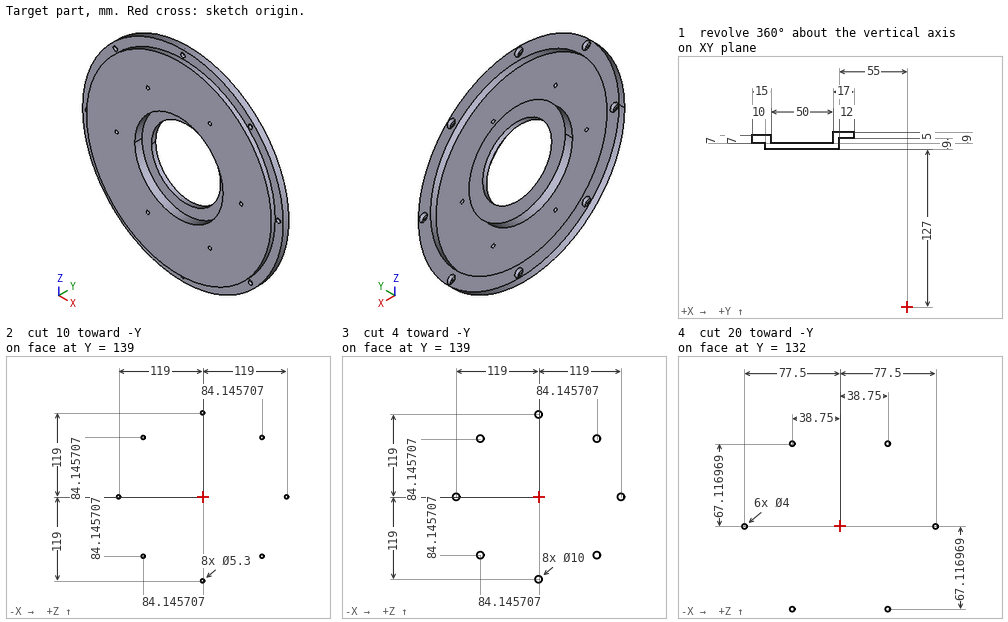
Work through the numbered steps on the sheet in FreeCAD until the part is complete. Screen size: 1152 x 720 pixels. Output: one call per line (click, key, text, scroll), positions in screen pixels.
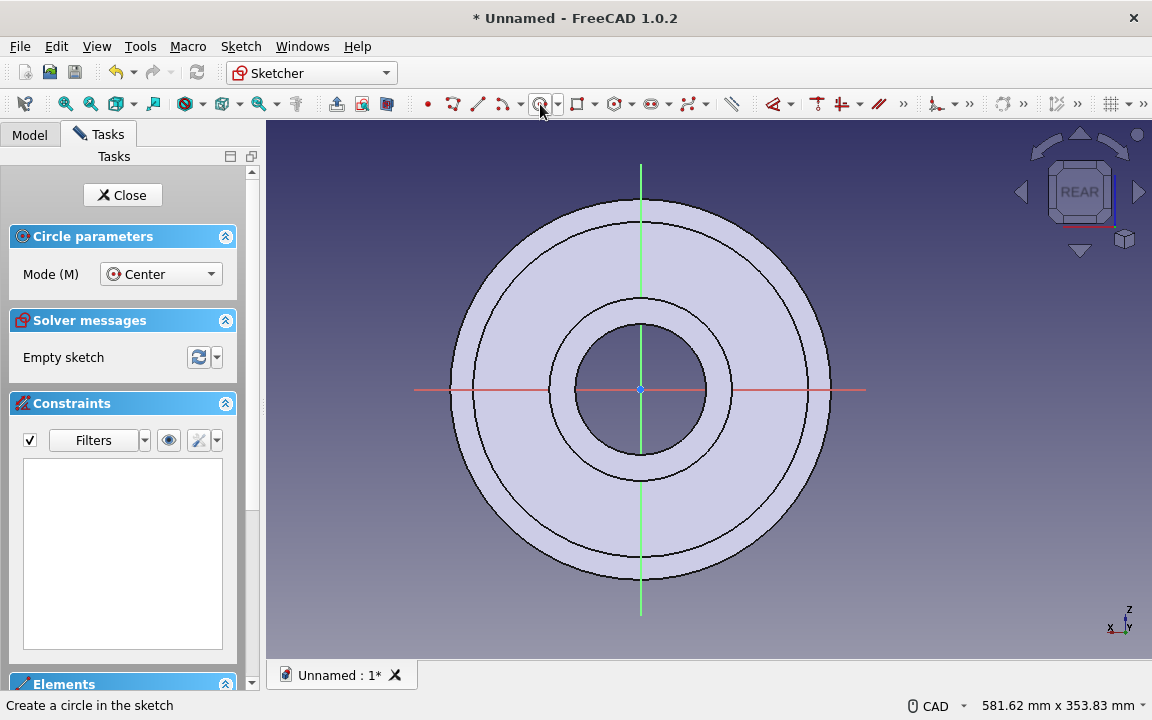
scroll(641, 571, up, 9)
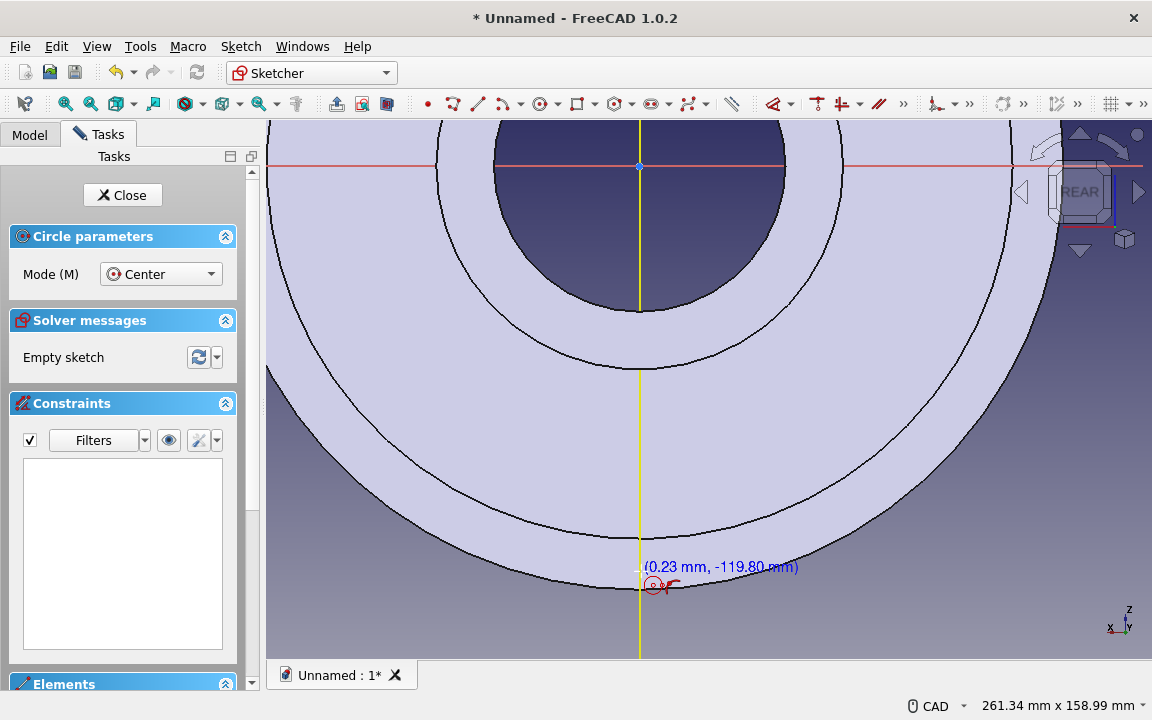
scroll(641, 572, down, 9)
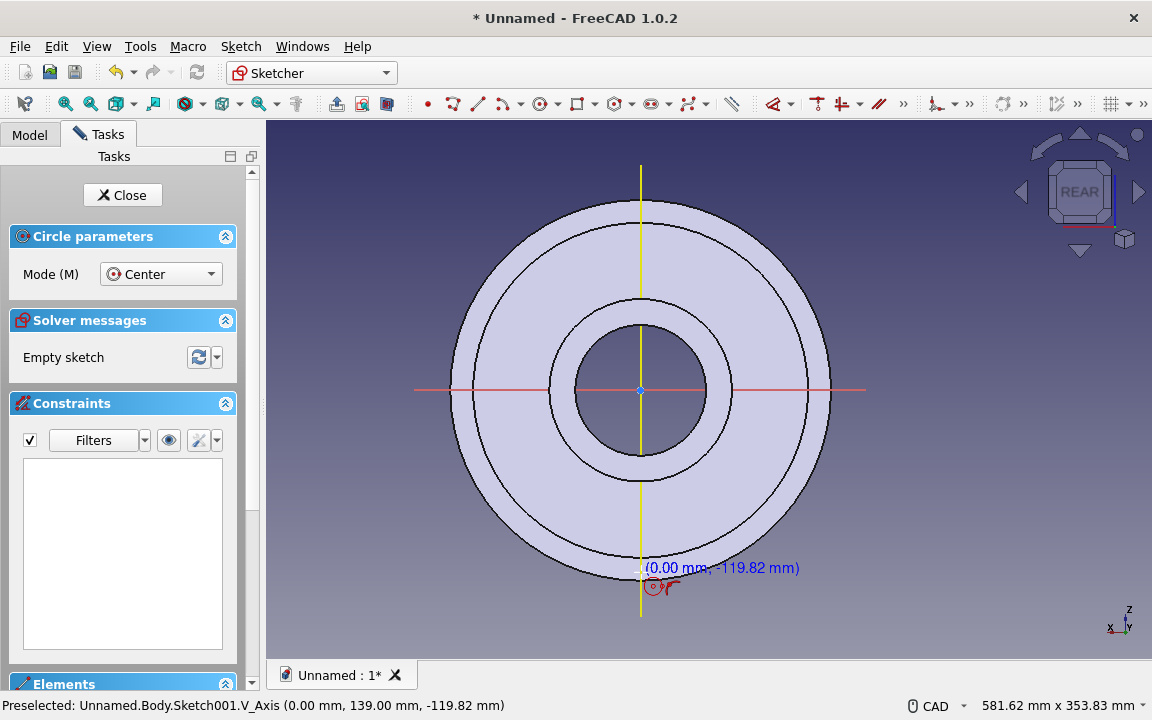
click(641, 572)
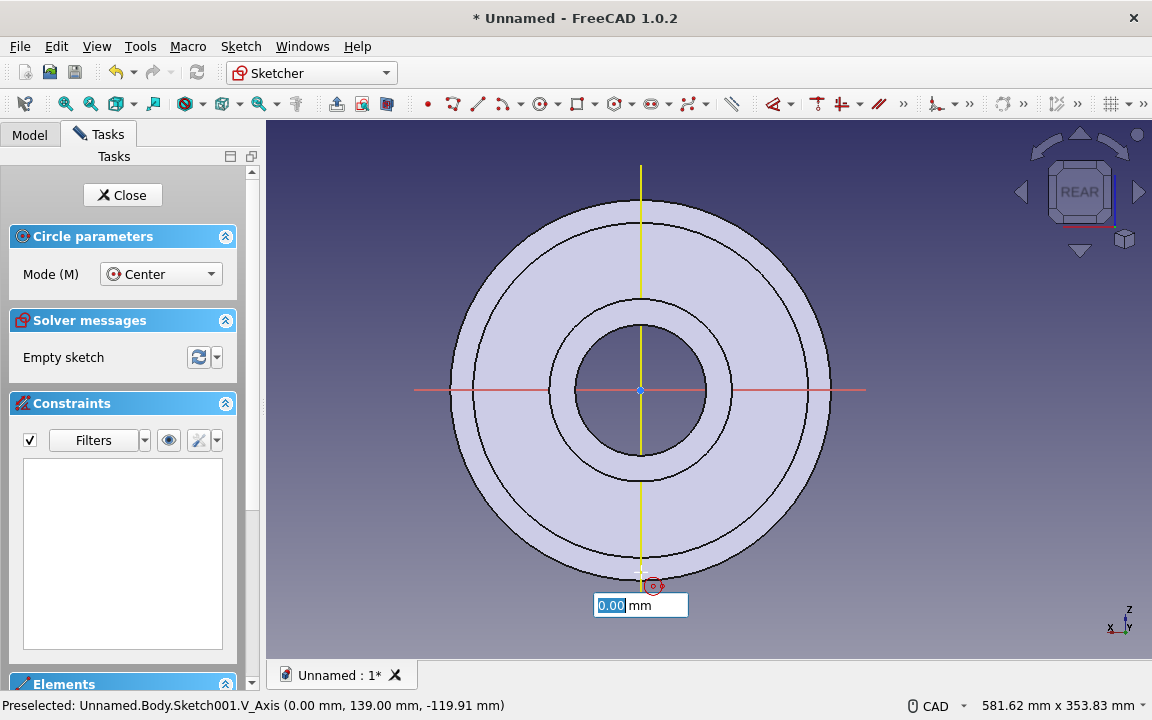
scroll(644, 570, up, 8)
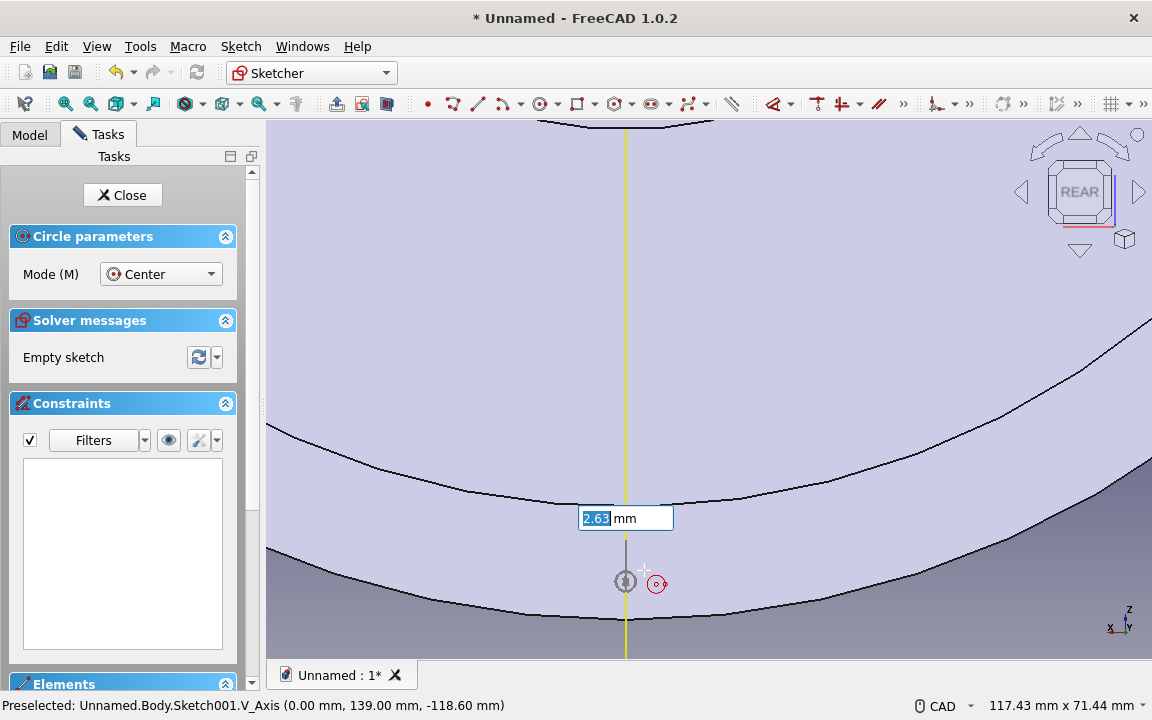
click(645, 568)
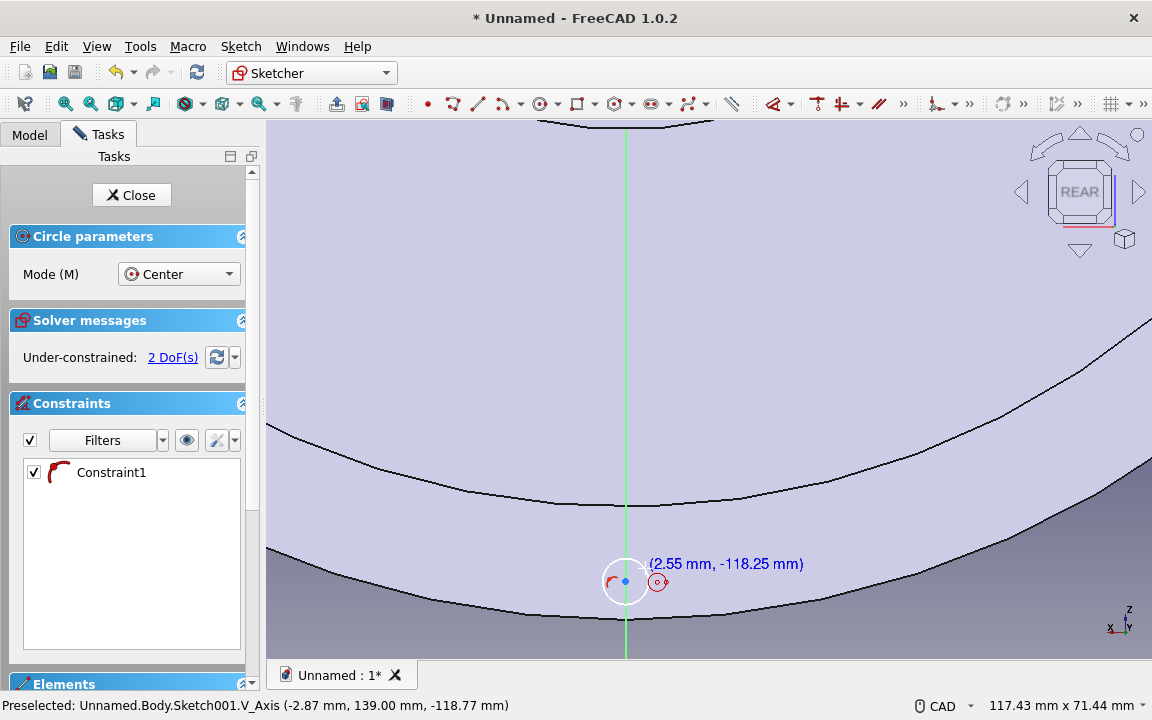
scroll(644, 570, down, 8)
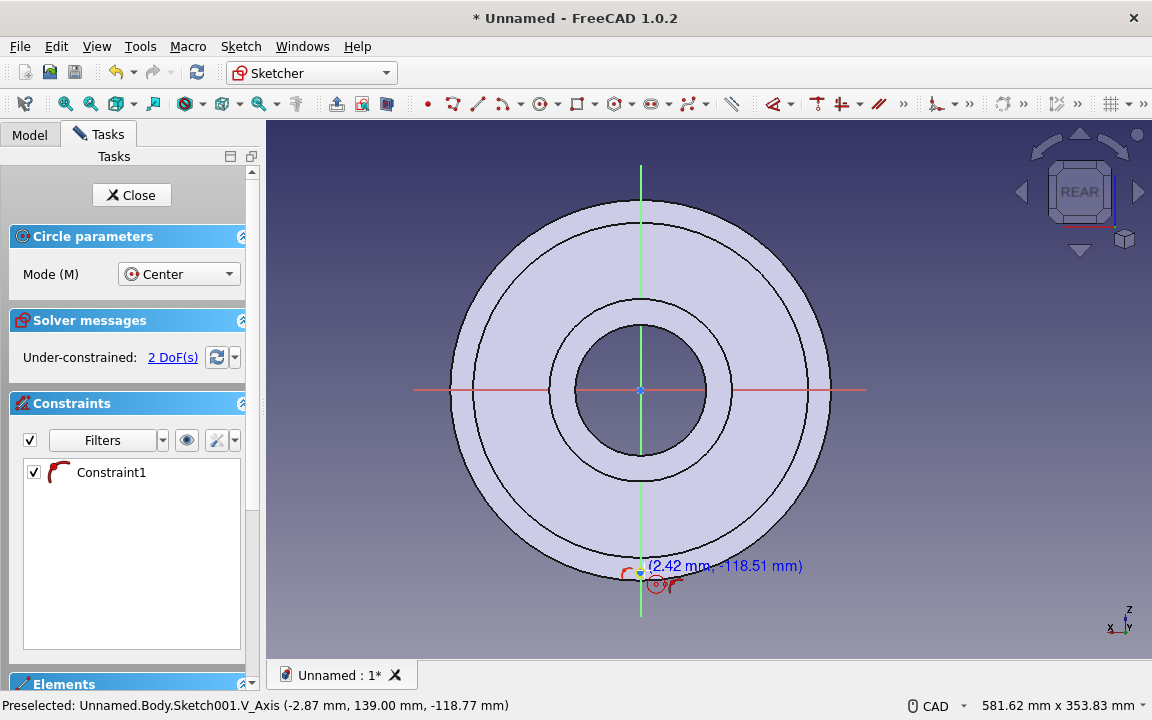
scroll(512, 519, up, 9)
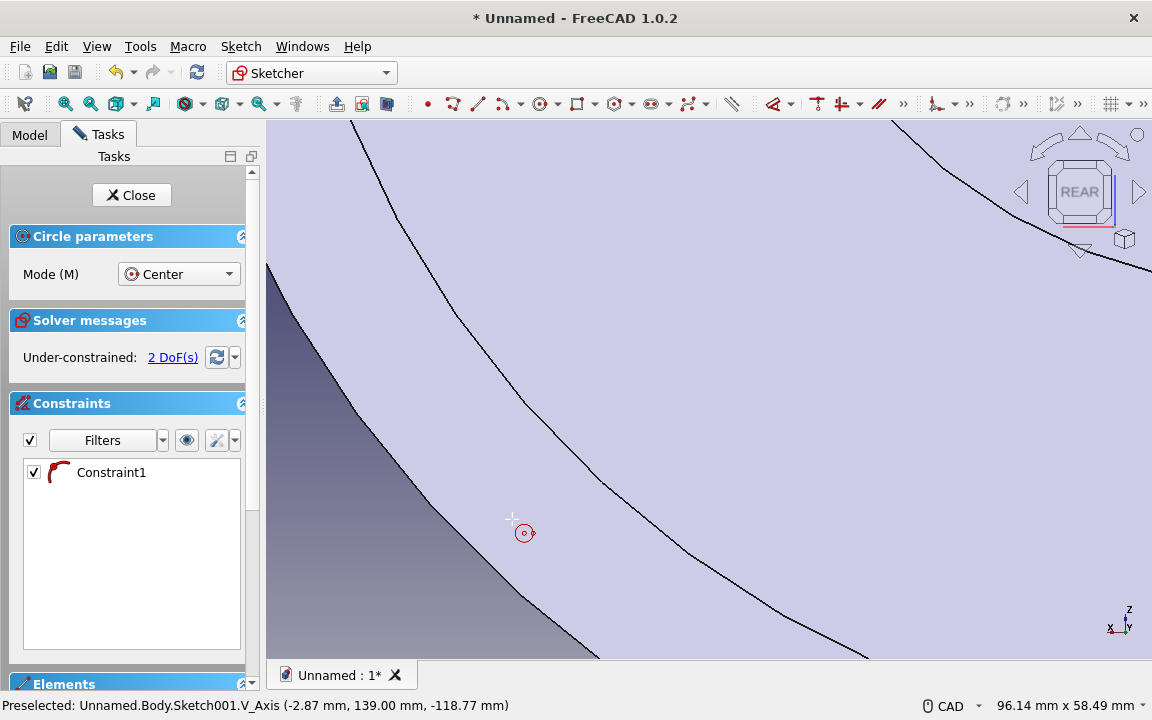
scroll(512, 519, down, 9)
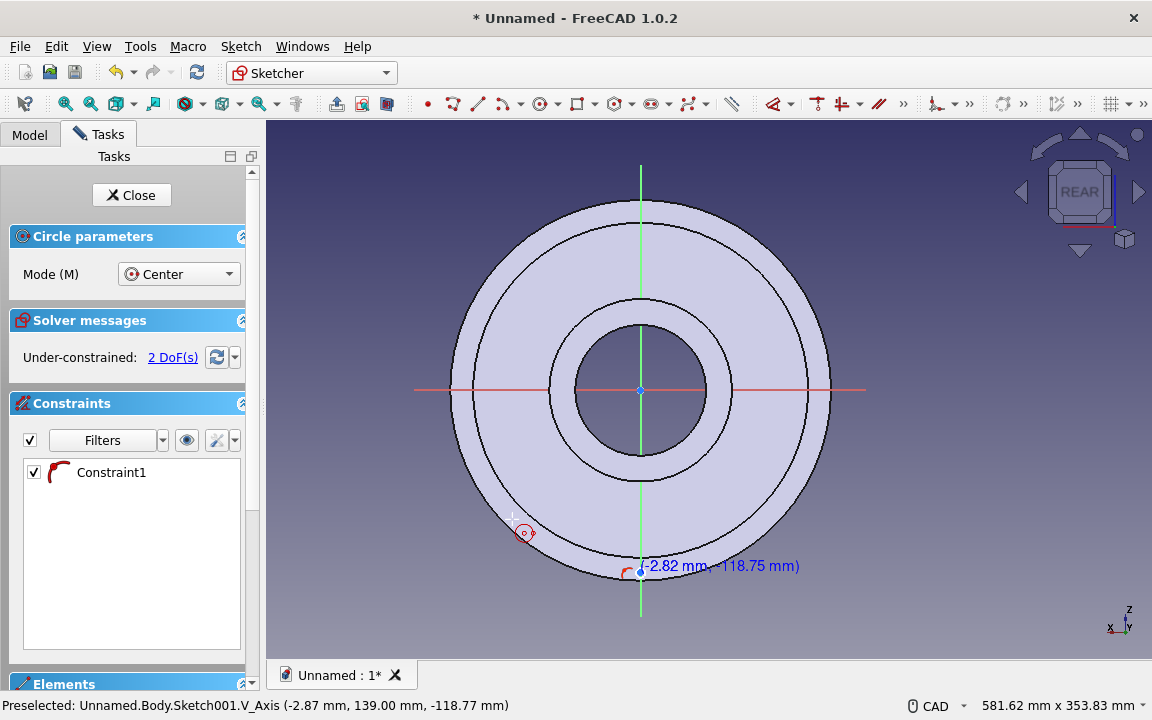
click(512, 519)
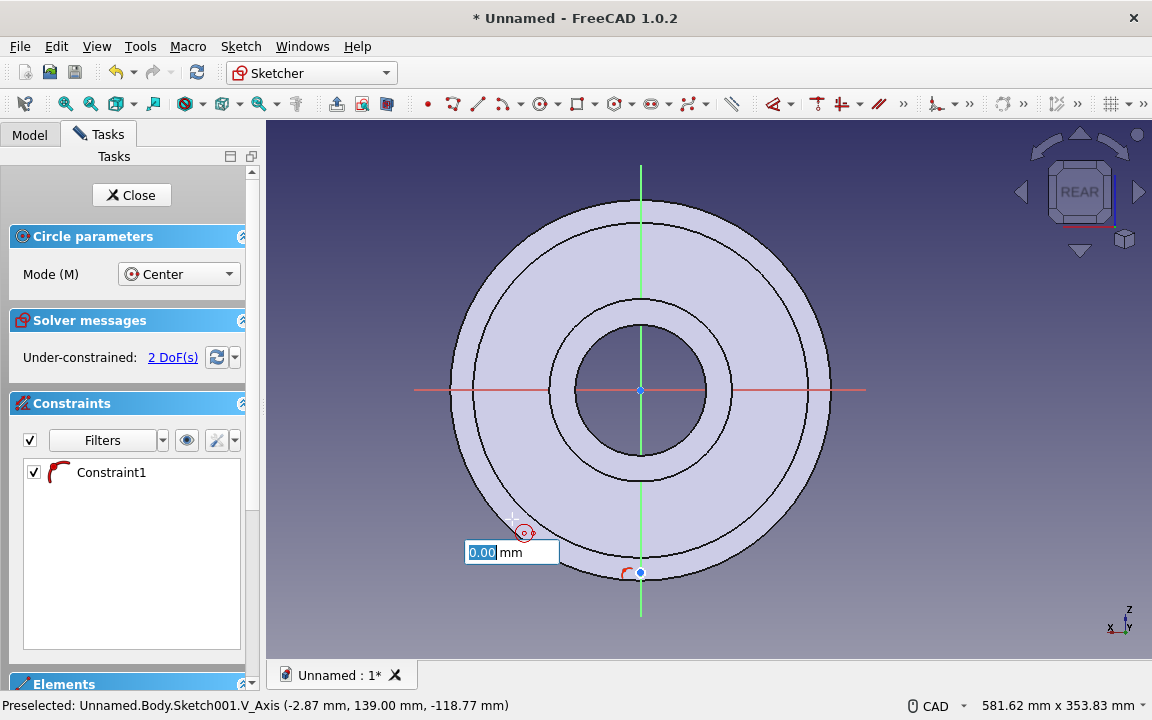
scroll(515, 516, up, 7)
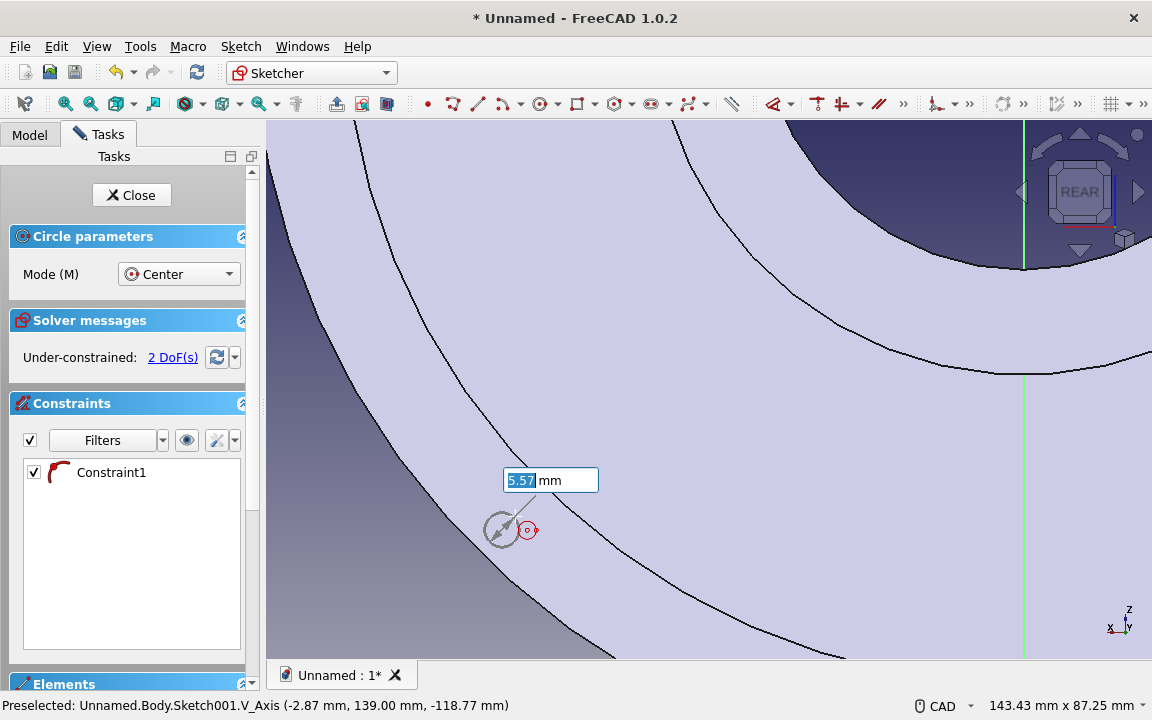
click(515, 512)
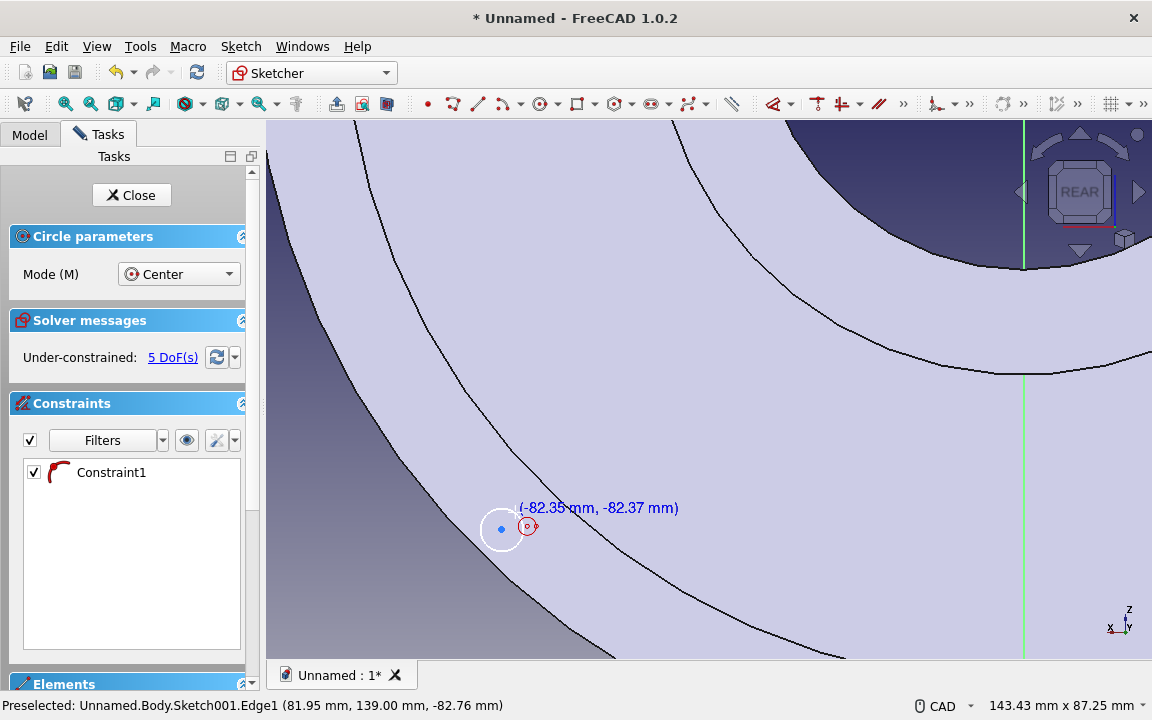
scroll(515, 516, down, 7)